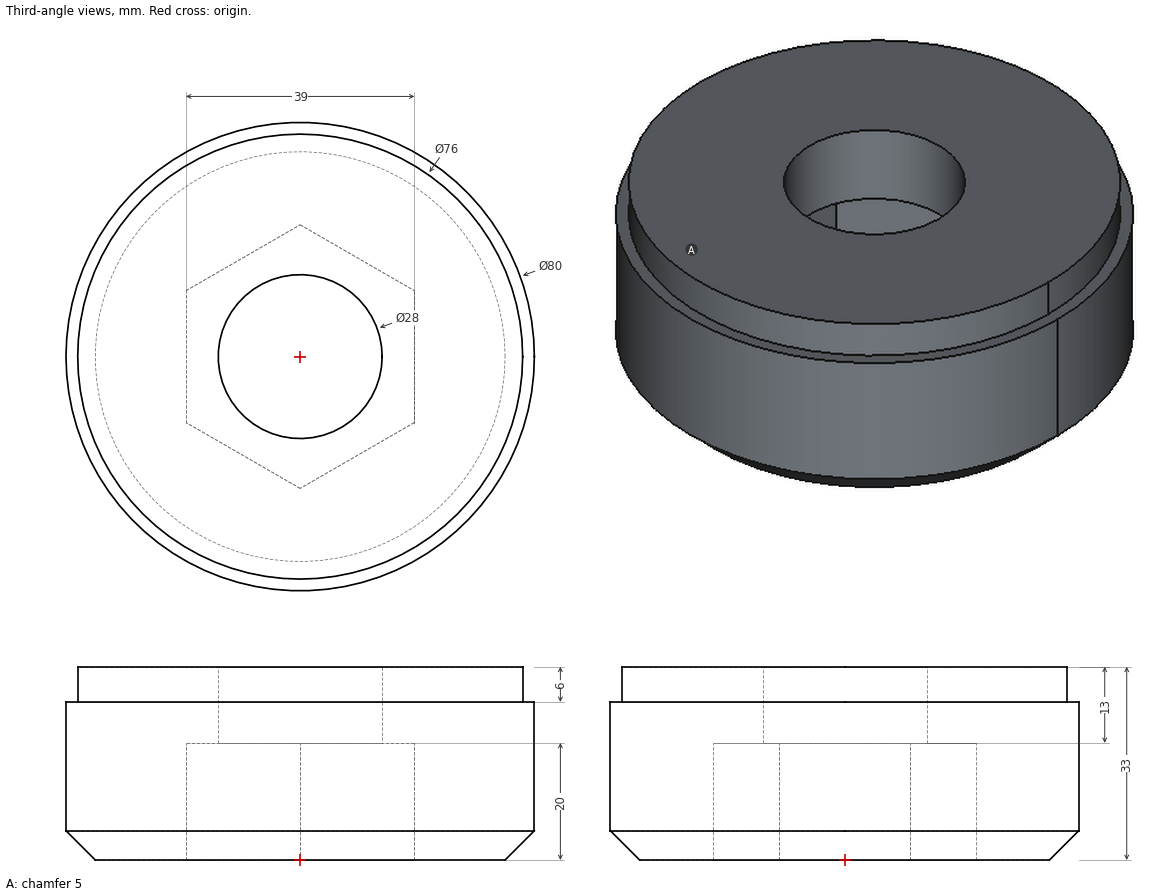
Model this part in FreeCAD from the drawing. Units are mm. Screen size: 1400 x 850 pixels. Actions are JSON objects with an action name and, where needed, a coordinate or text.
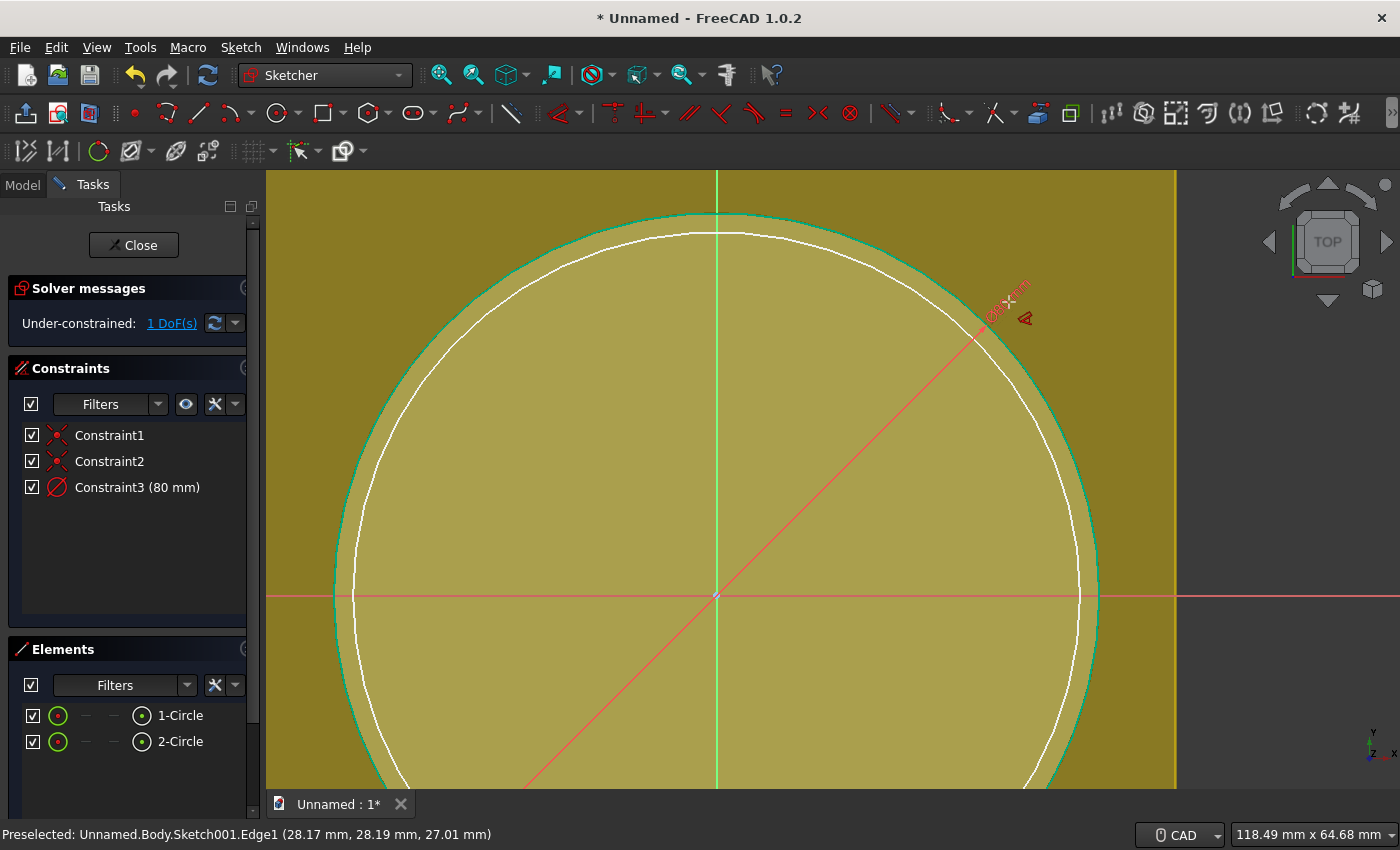
{"action": "left_click", "coordinate": [973, 338]}
{"action": "left_click", "coordinate": [1118, 477]}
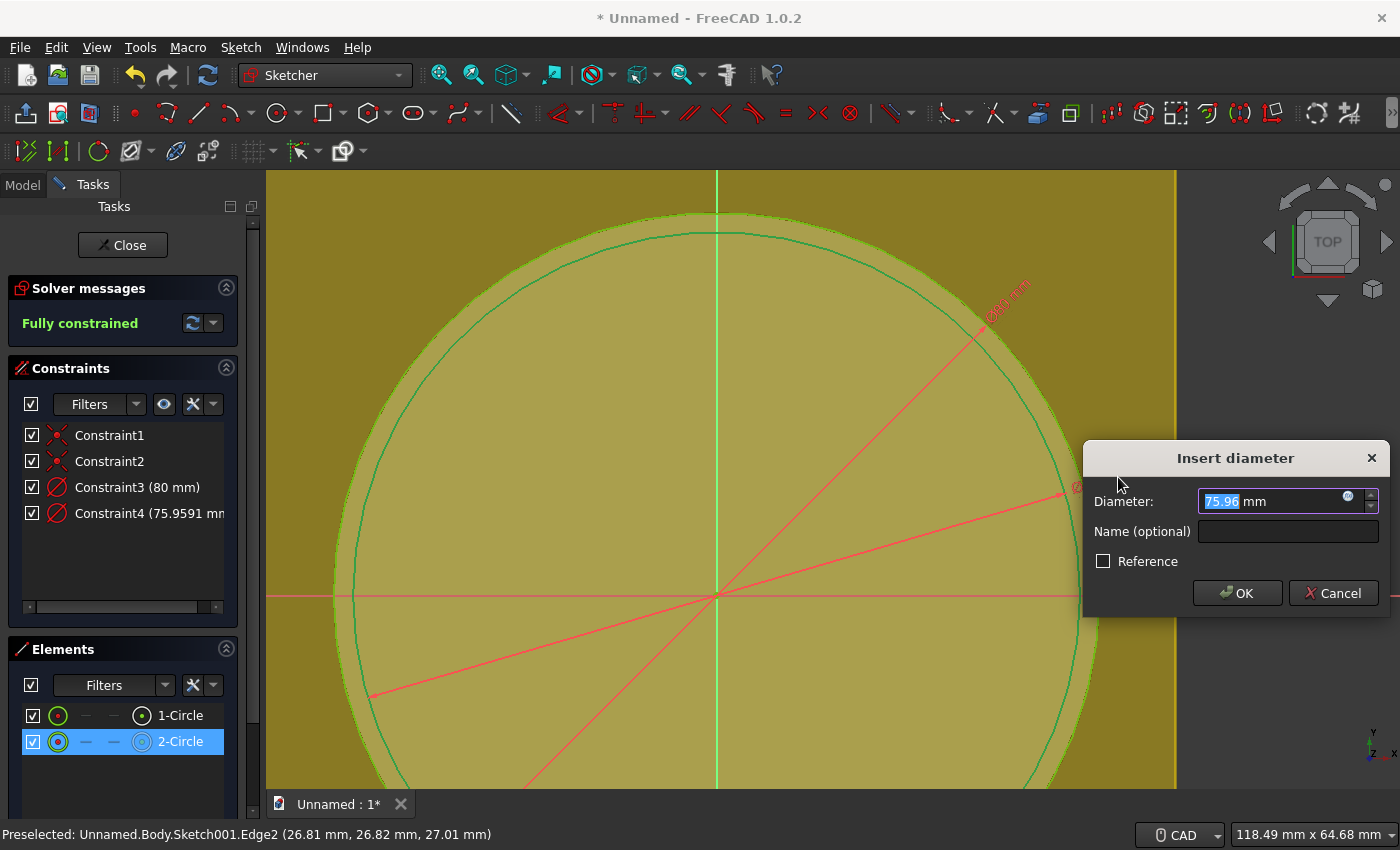
{"action": "type", "text": "76"}
{"action": "key", "text": "Return"}
{"action": "key", "text": "Escape"}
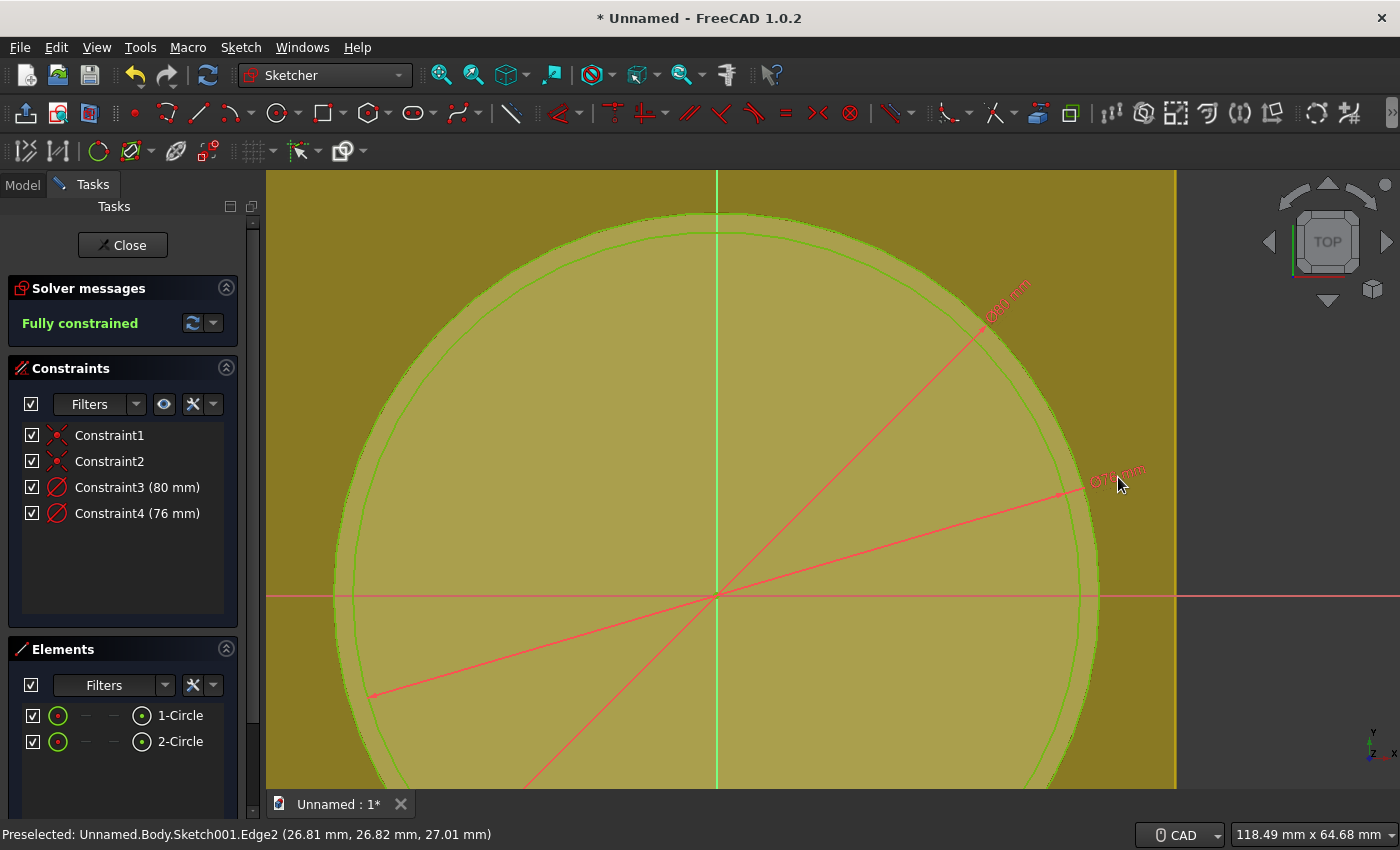
{"action": "left_click", "coordinate": [123, 245]}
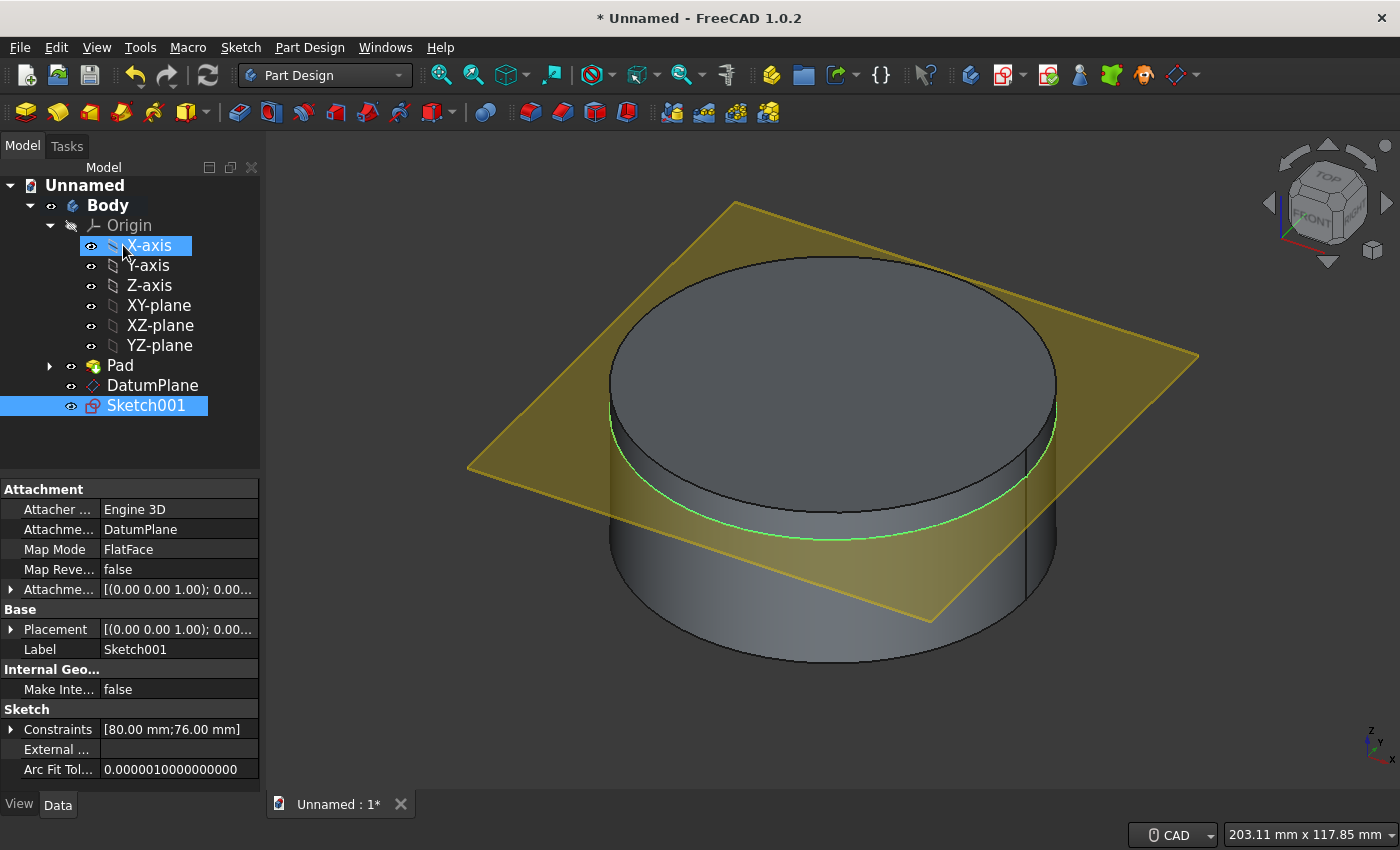
{"action": "left_click", "coordinate": [240, 112]}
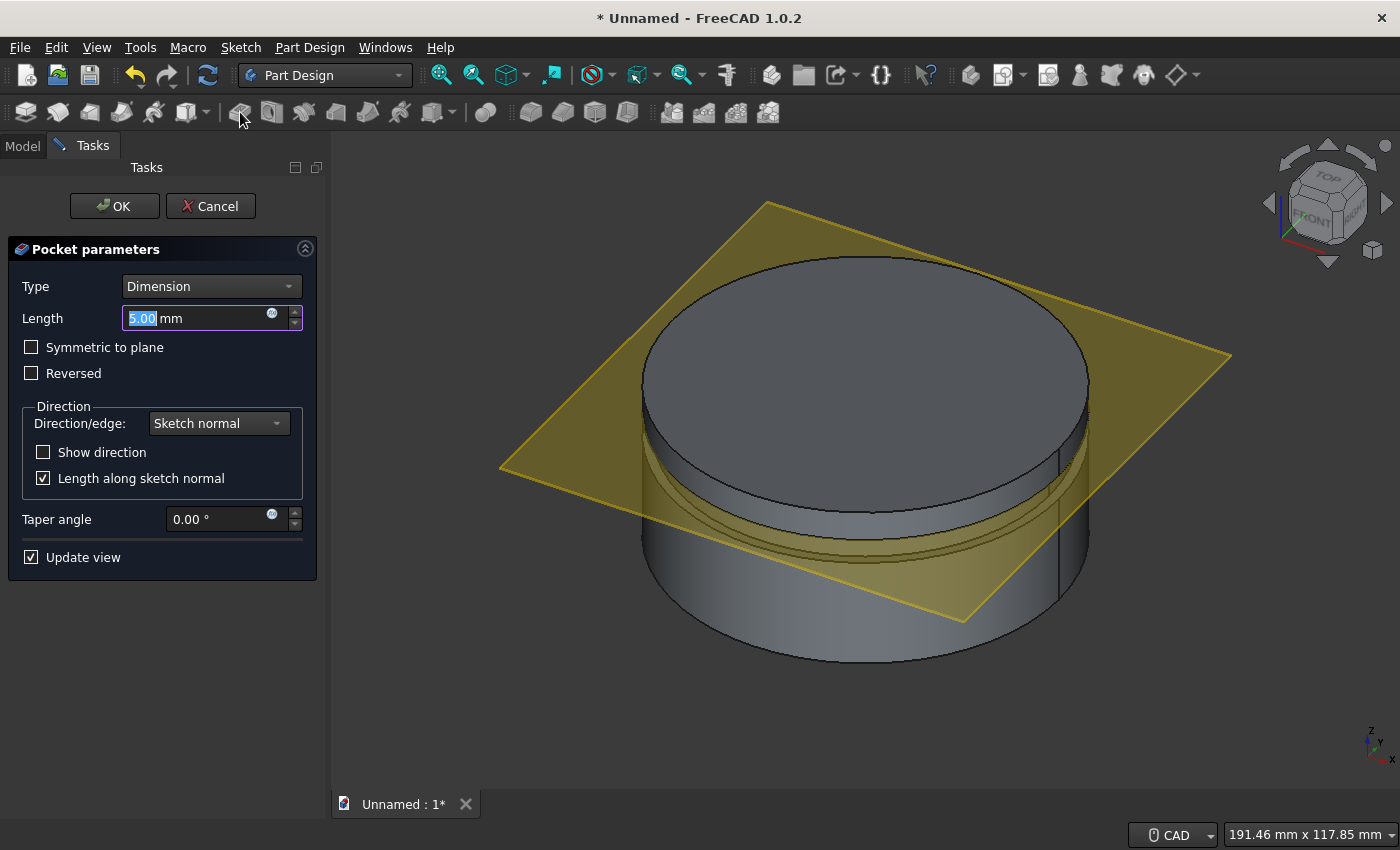
{"action": "type", "text": "6"}
{"action": "key", "text": "Tab"}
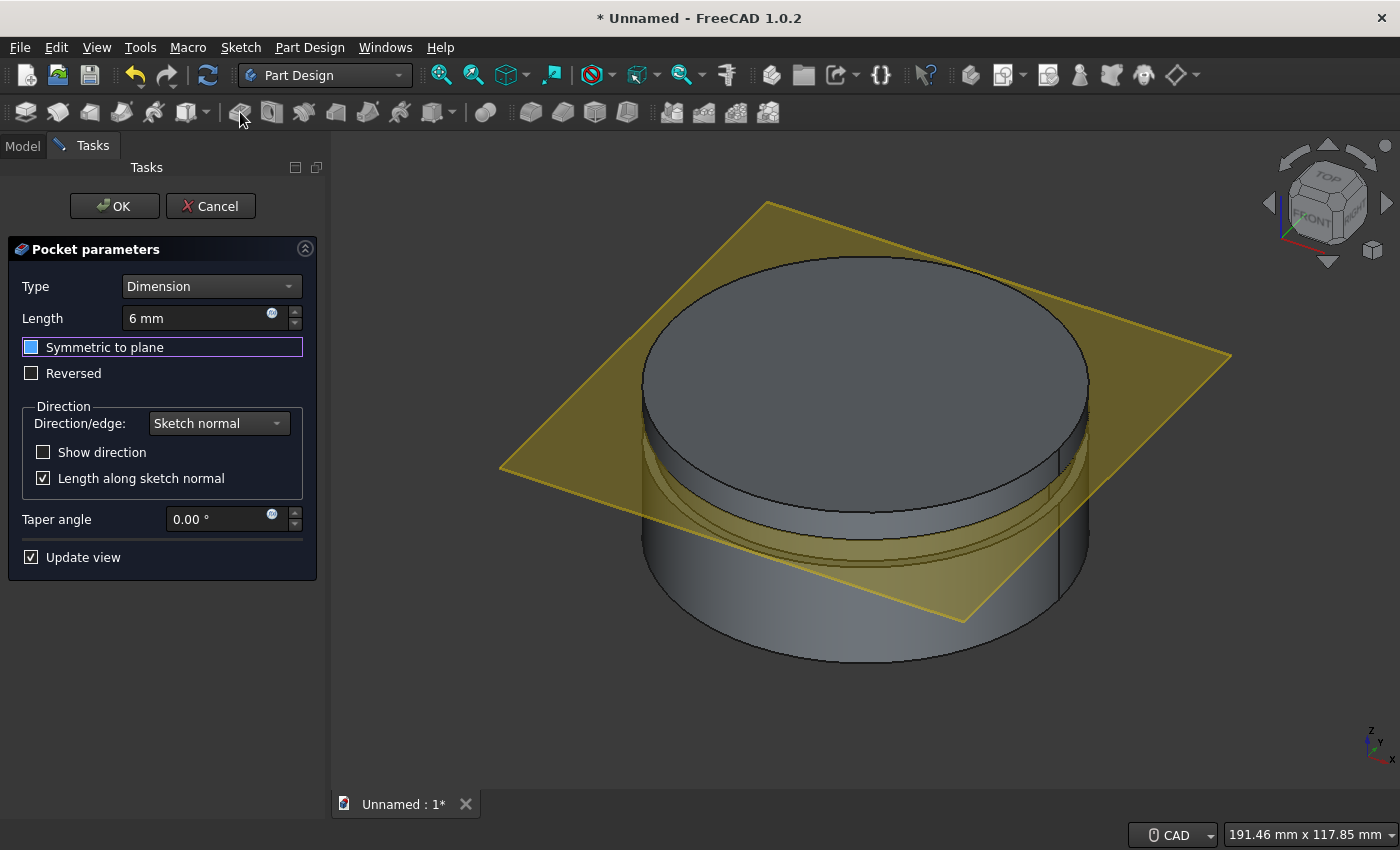
{"action": "left_click", "coordinate": [30, 373]}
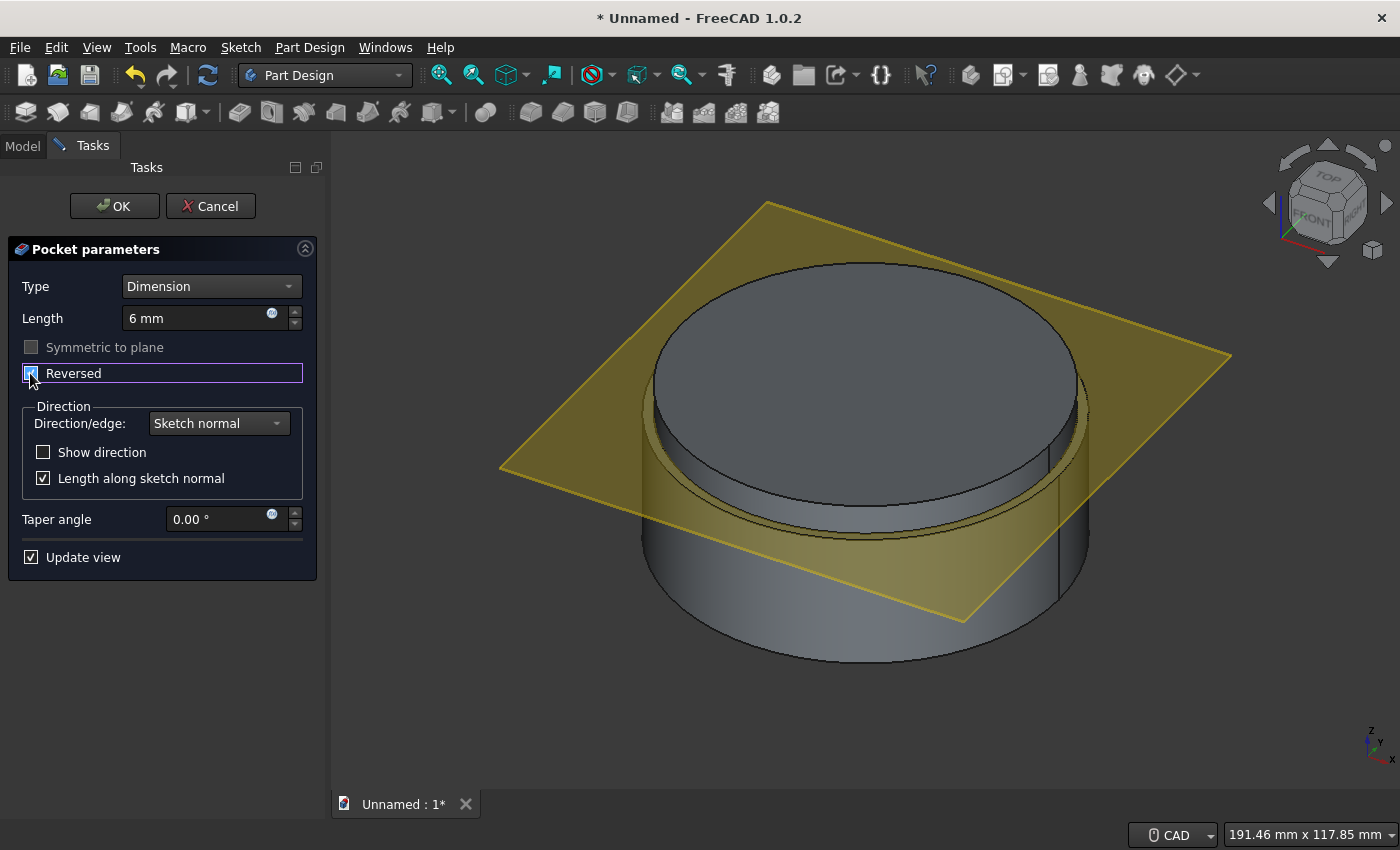
{"action": "left_click", "coordinate": [115, 206]}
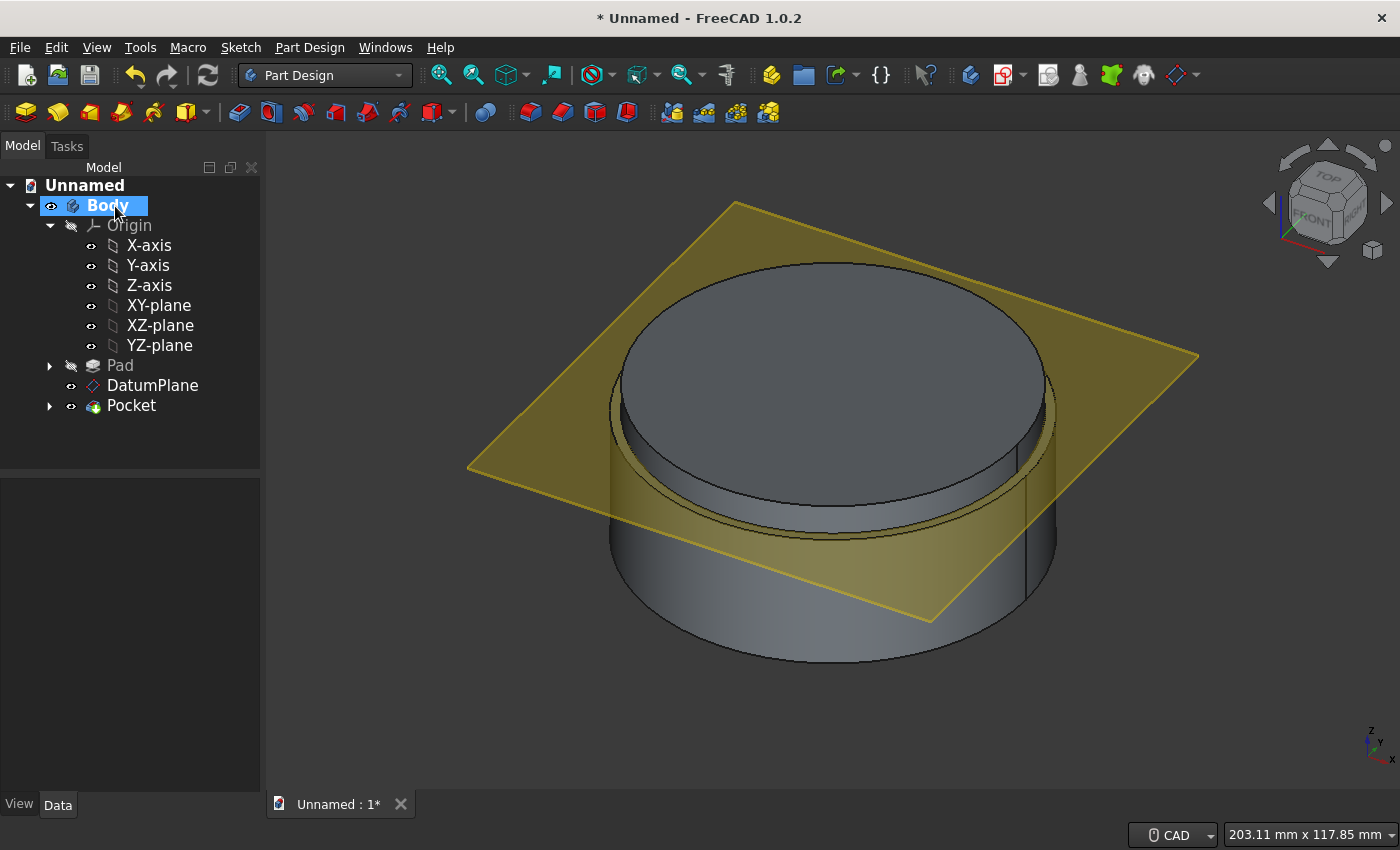
{"action": "left_click", "coordinate": [116, 386]}
{"action": "key", "text": "space"}